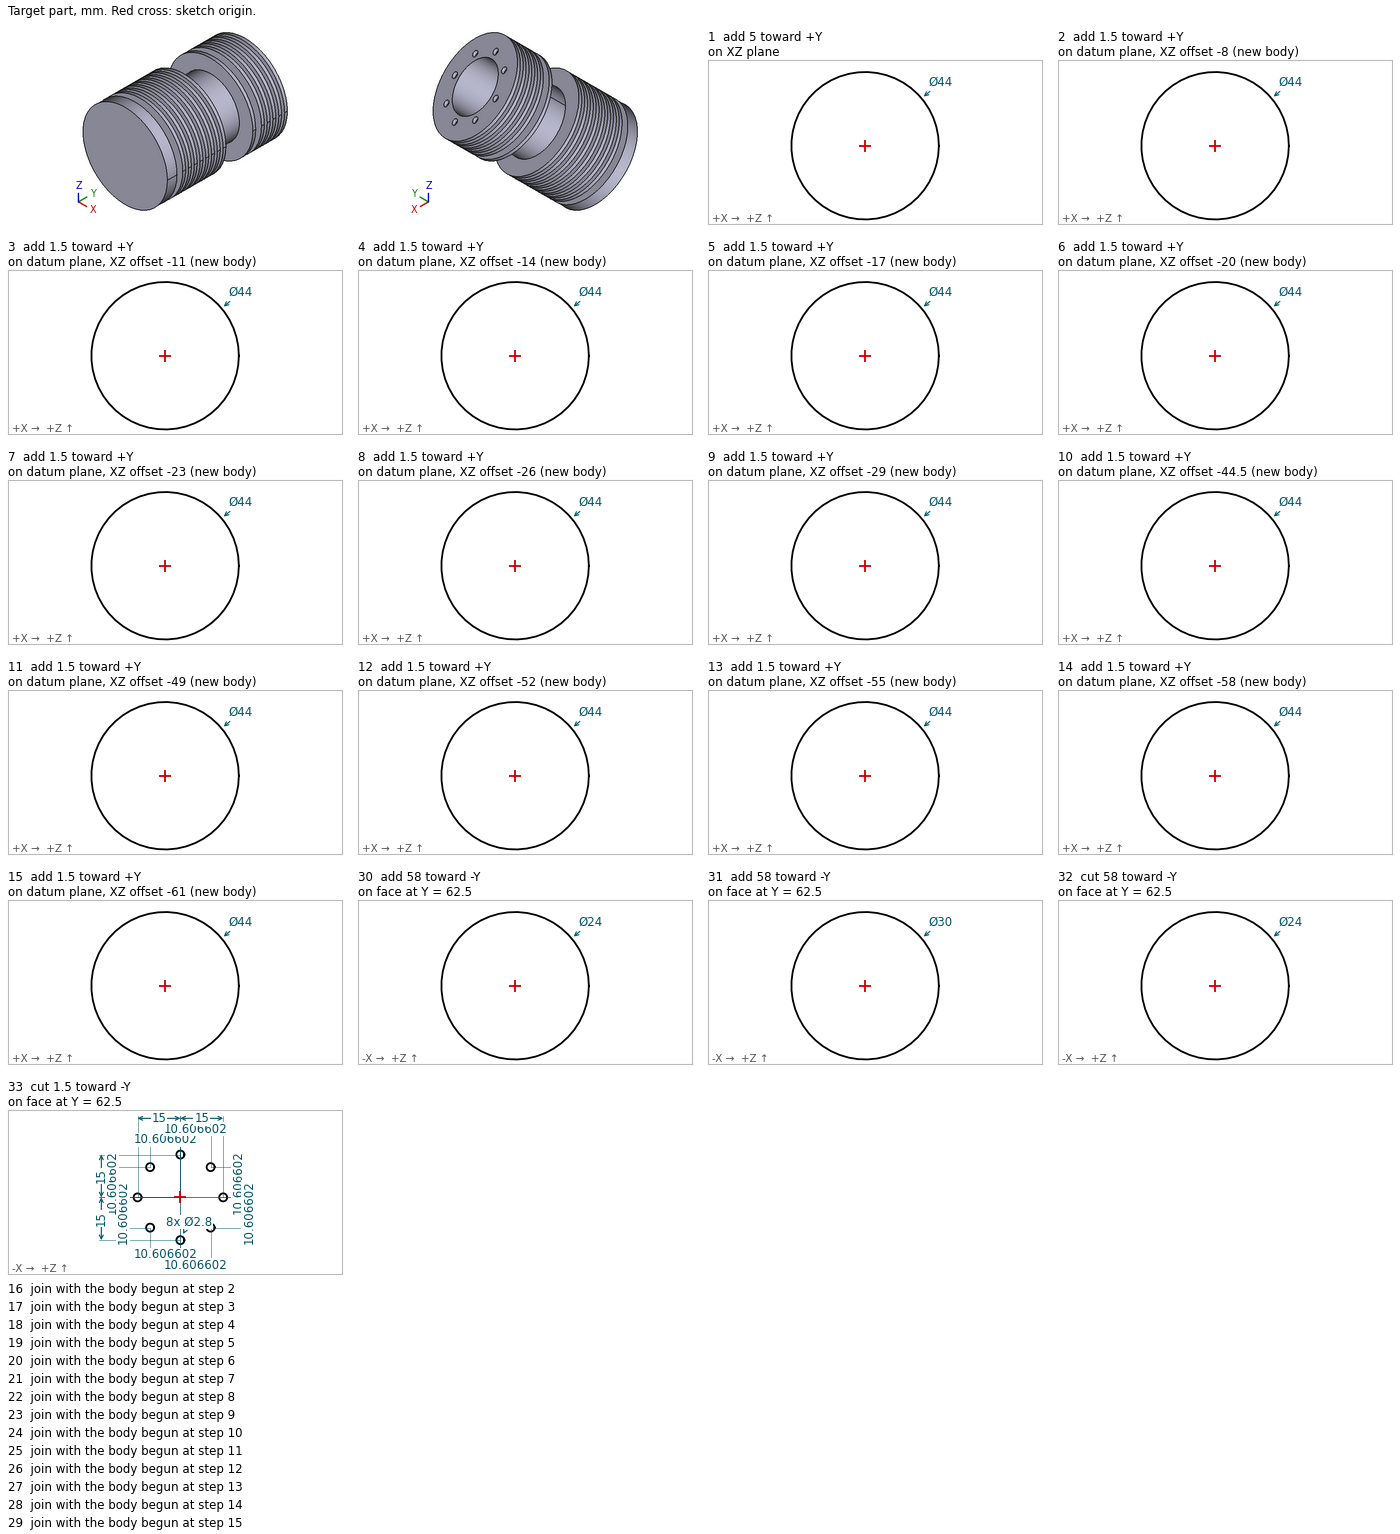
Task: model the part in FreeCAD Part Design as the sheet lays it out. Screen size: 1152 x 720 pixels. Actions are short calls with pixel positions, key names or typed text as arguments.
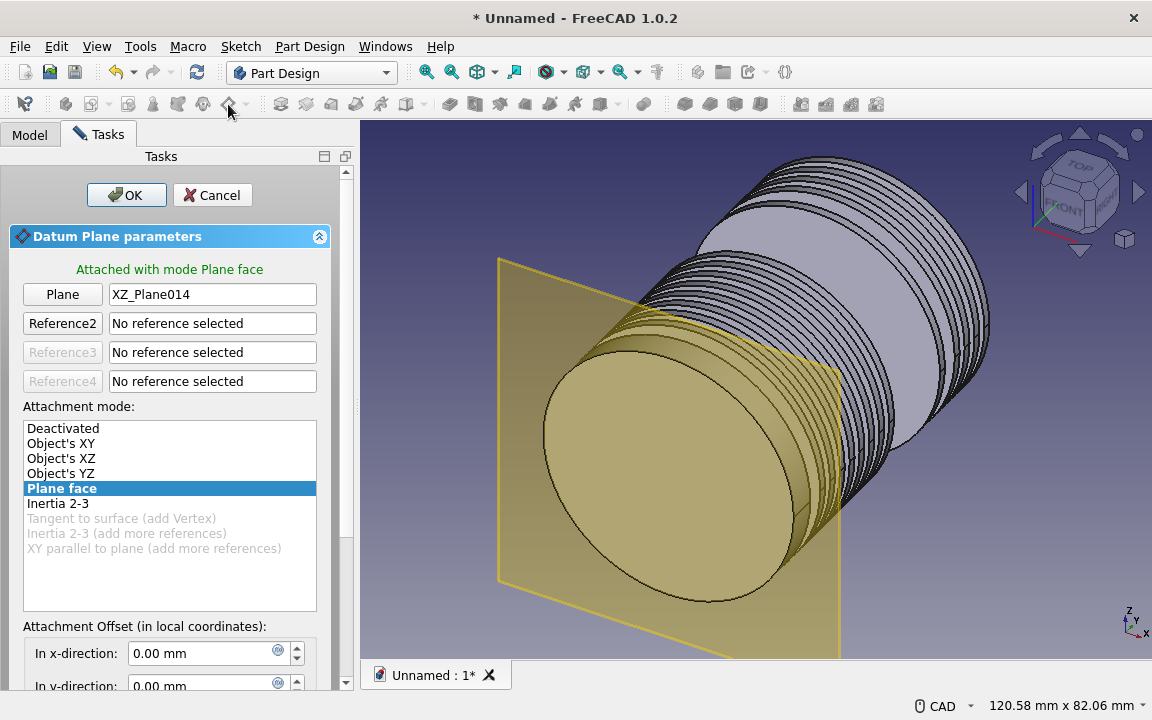
scroll(346, 428, down, 2)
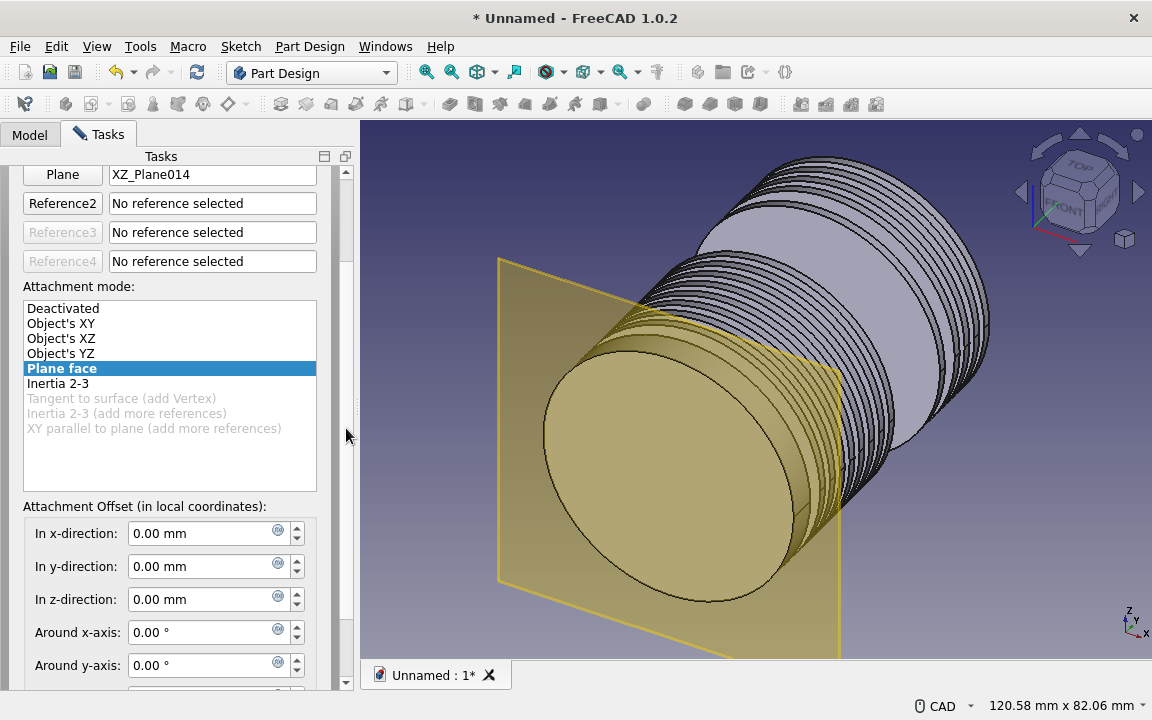
triple_click(210, 600)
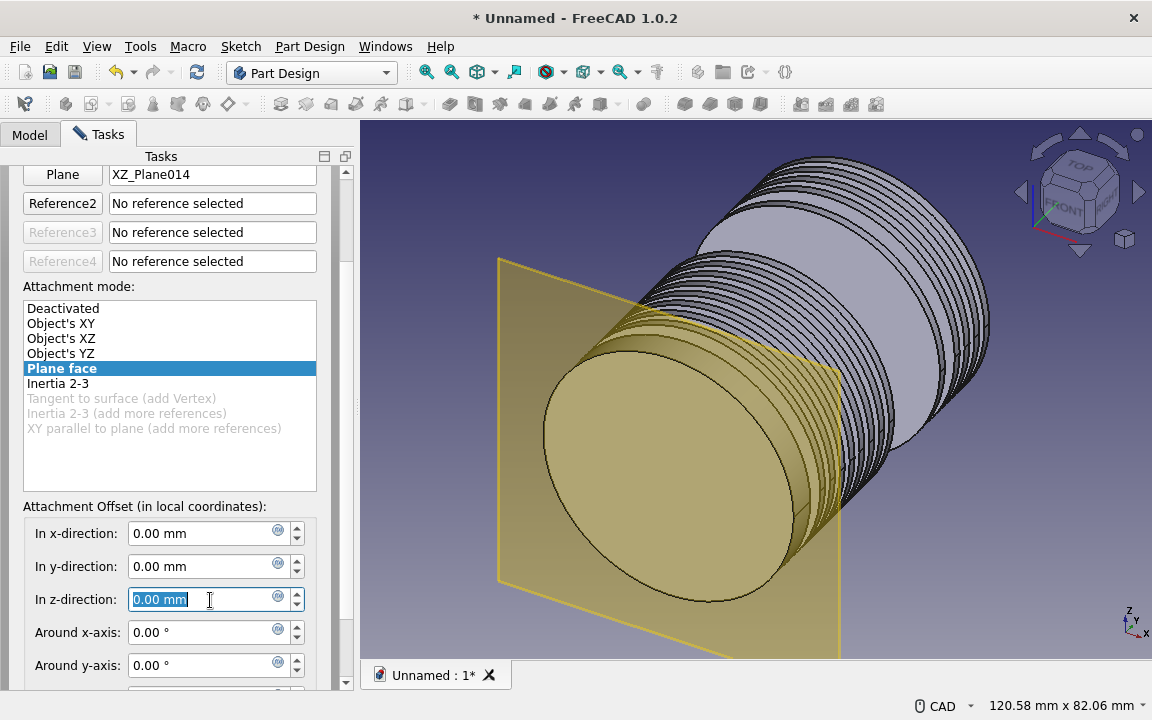
text(-61)
key(Tab)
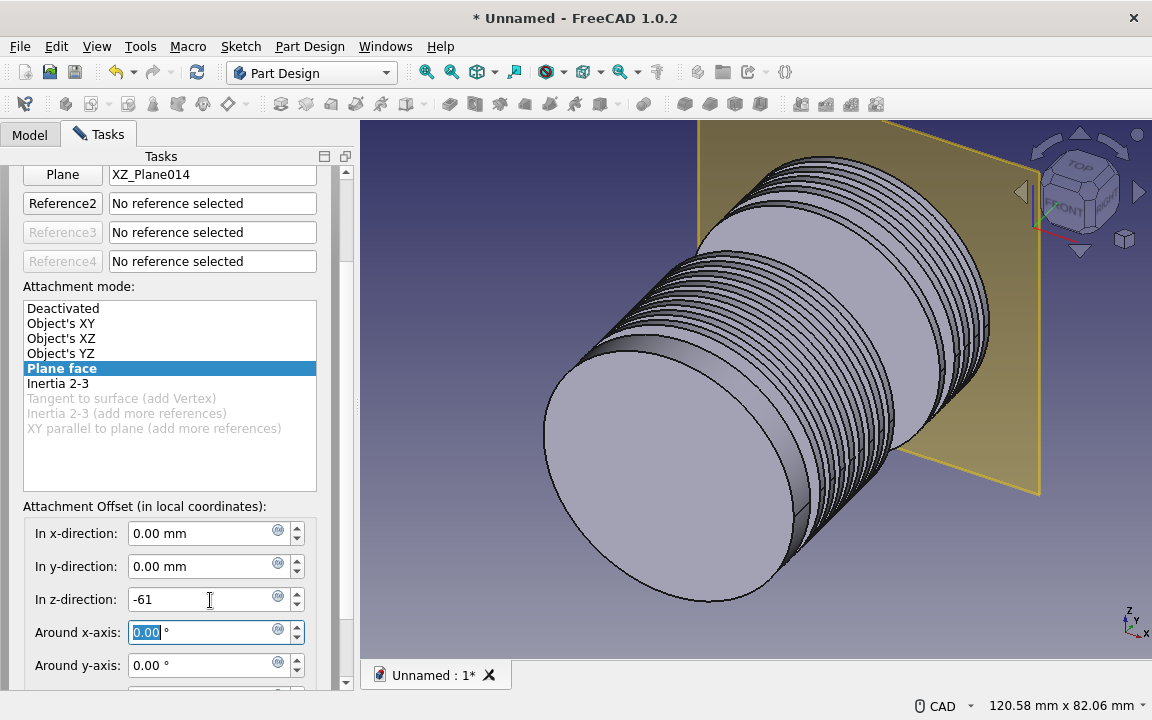
scroll(346, 428, up, 3)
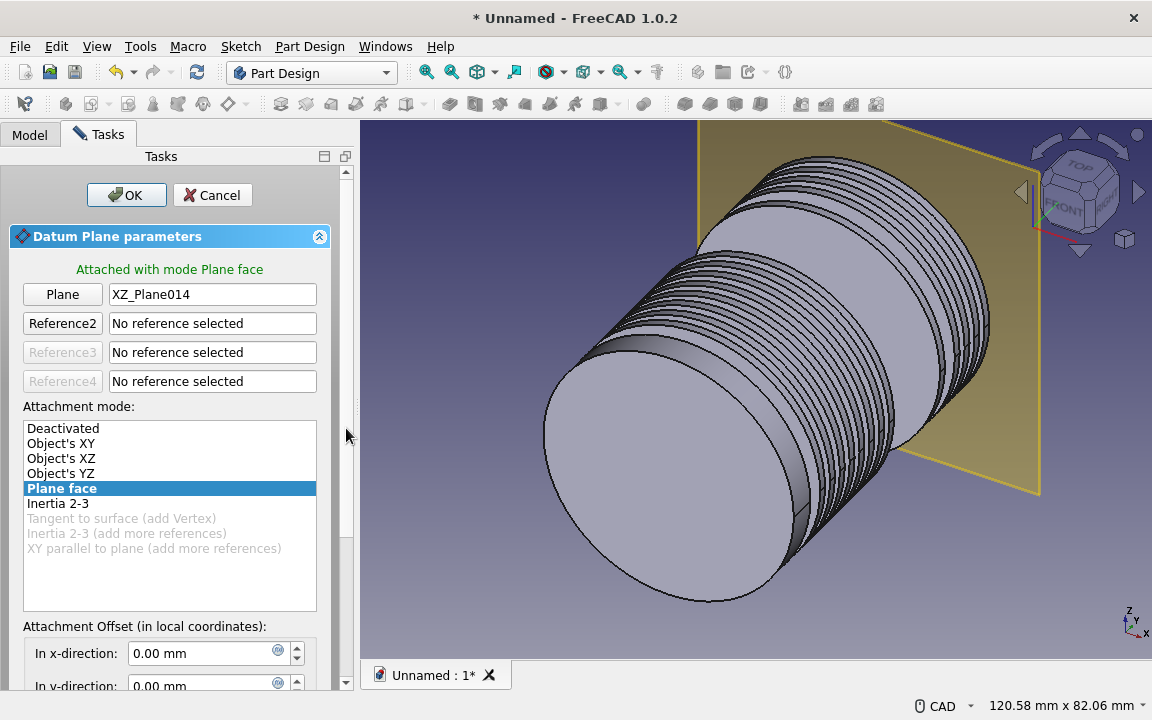
click(127, 195)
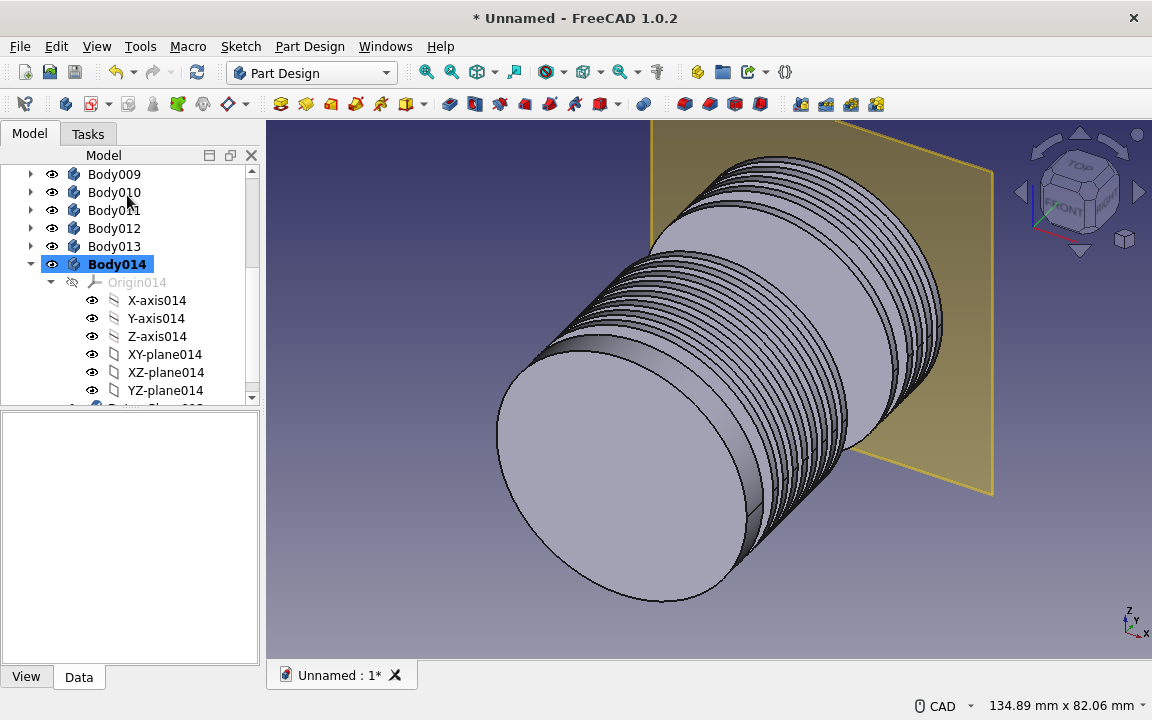
scroll(121, 278, down, 3)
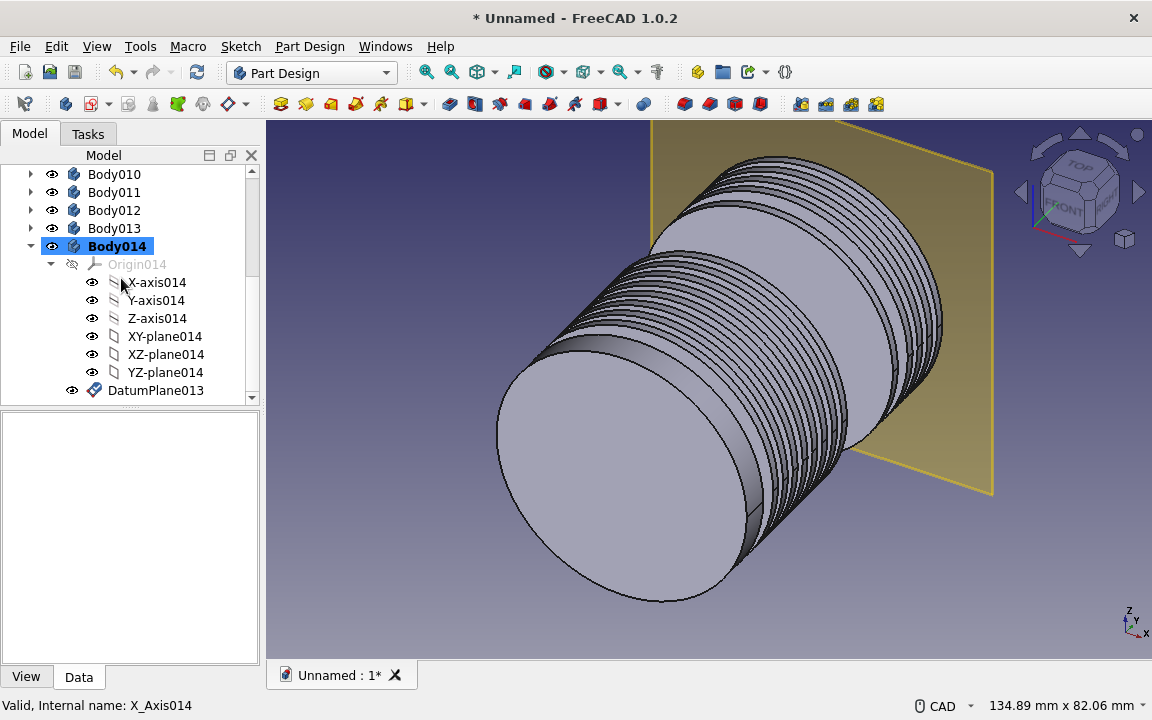
click(117, 390)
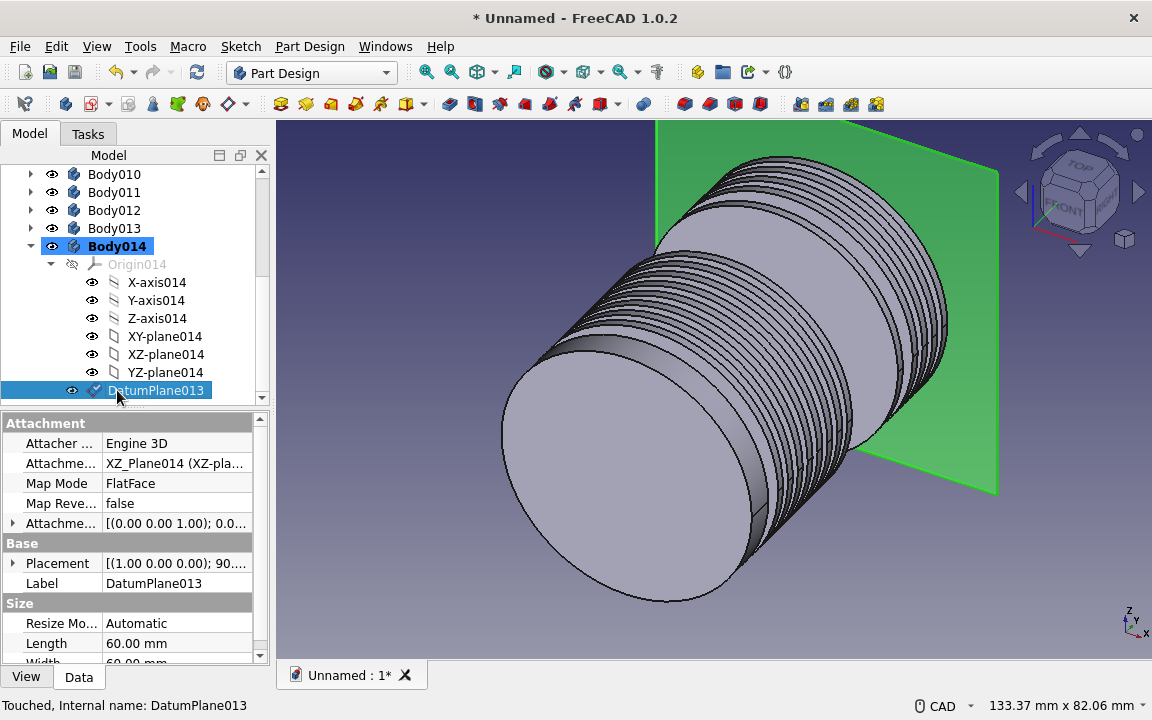
click(90, 104)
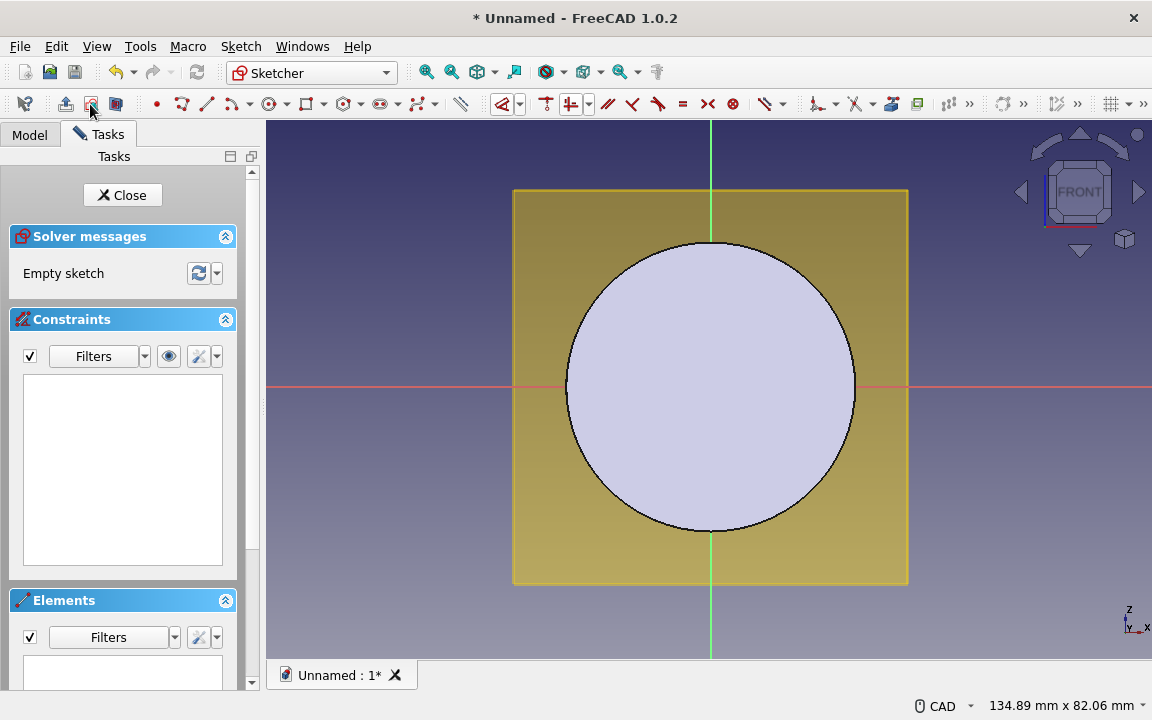
key(g)
key(c)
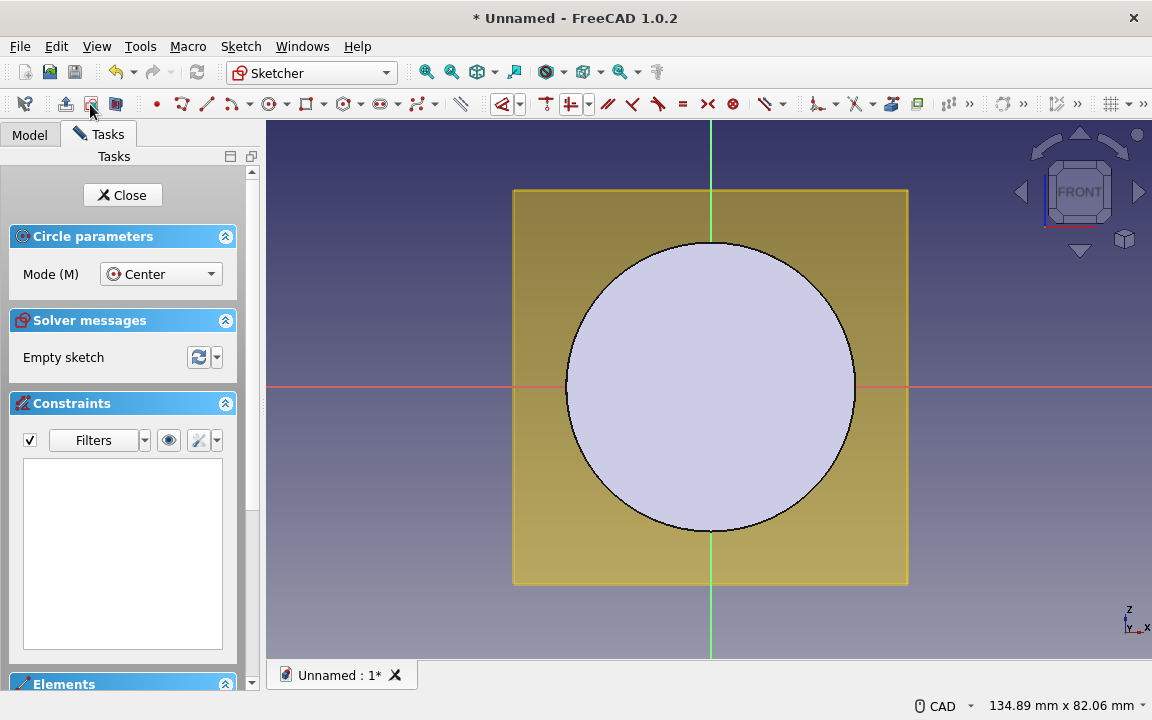
click(711, 387)
click(813, 285)
key(Escape)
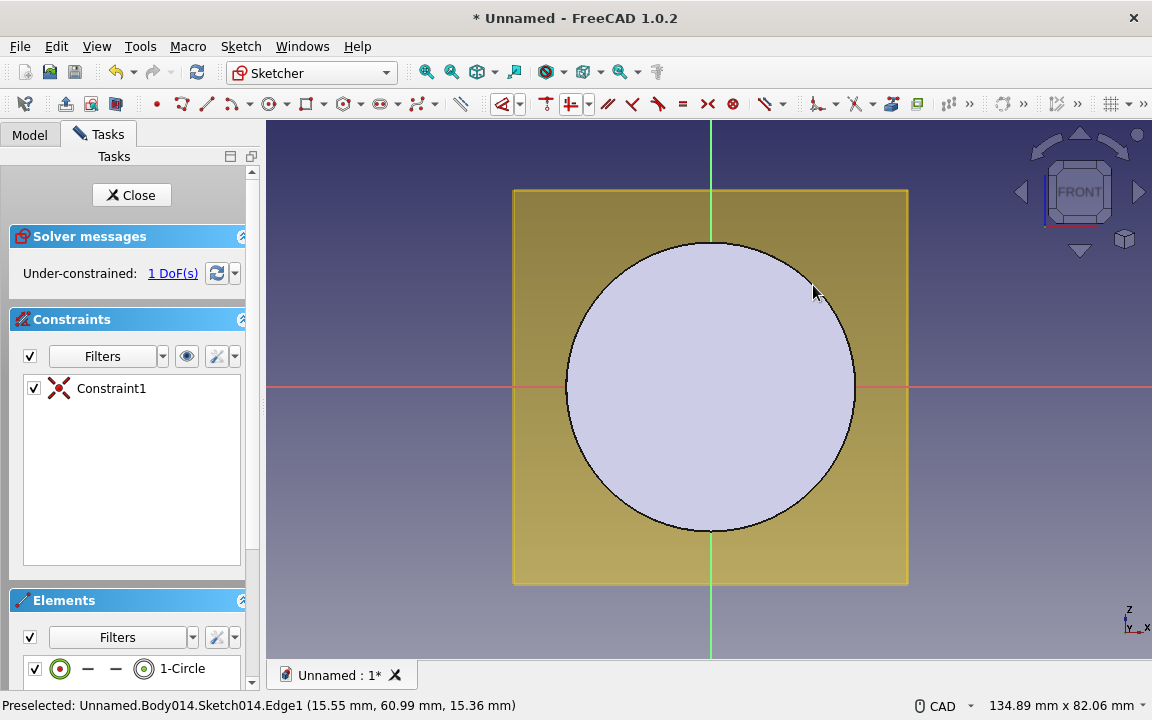
click(812, 285)